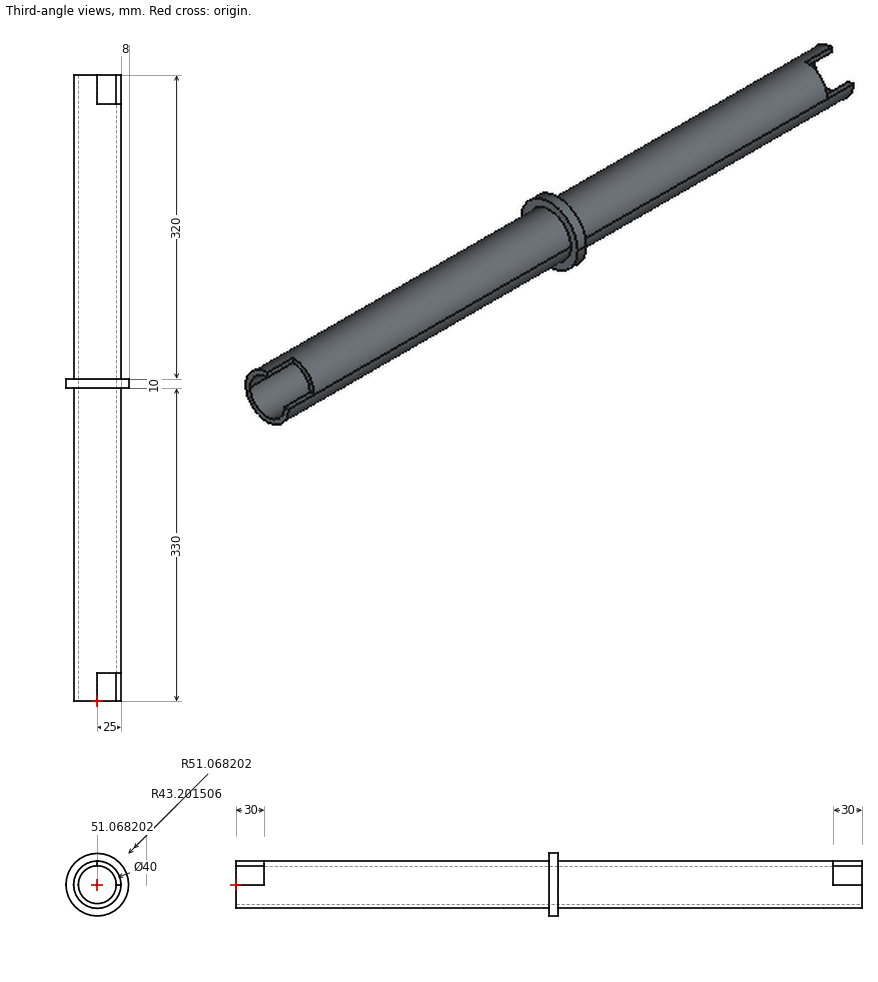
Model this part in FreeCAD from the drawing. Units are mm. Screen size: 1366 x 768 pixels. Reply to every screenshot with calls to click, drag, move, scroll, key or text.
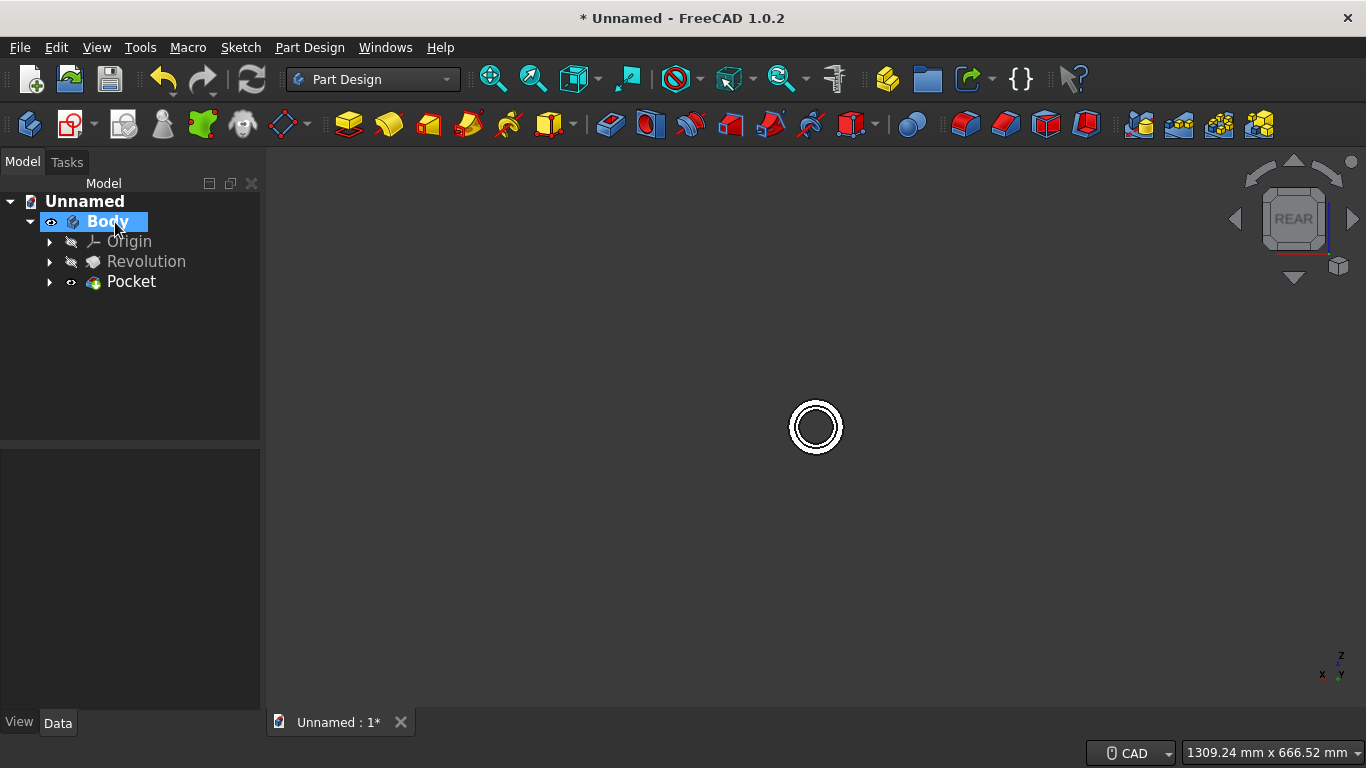
click(494, 80)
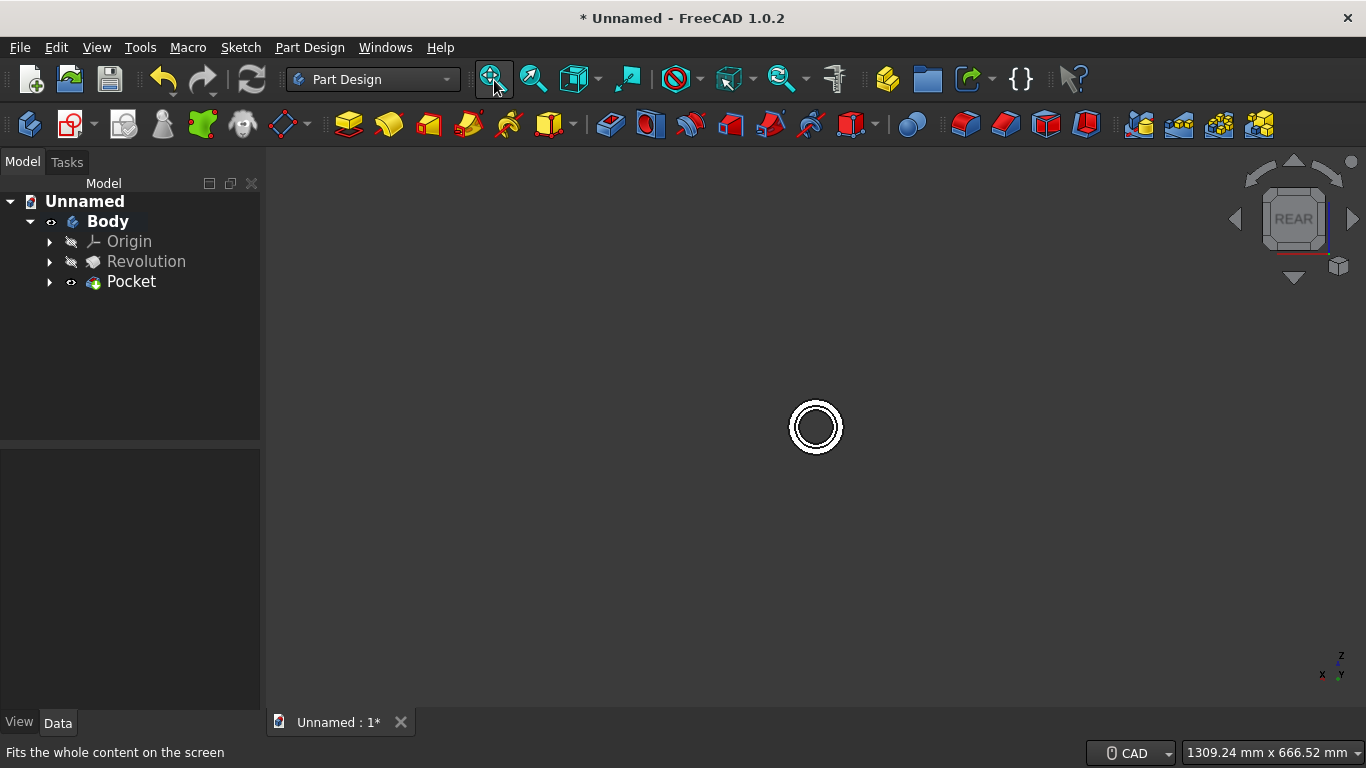
scroll(834, 432, up, 9)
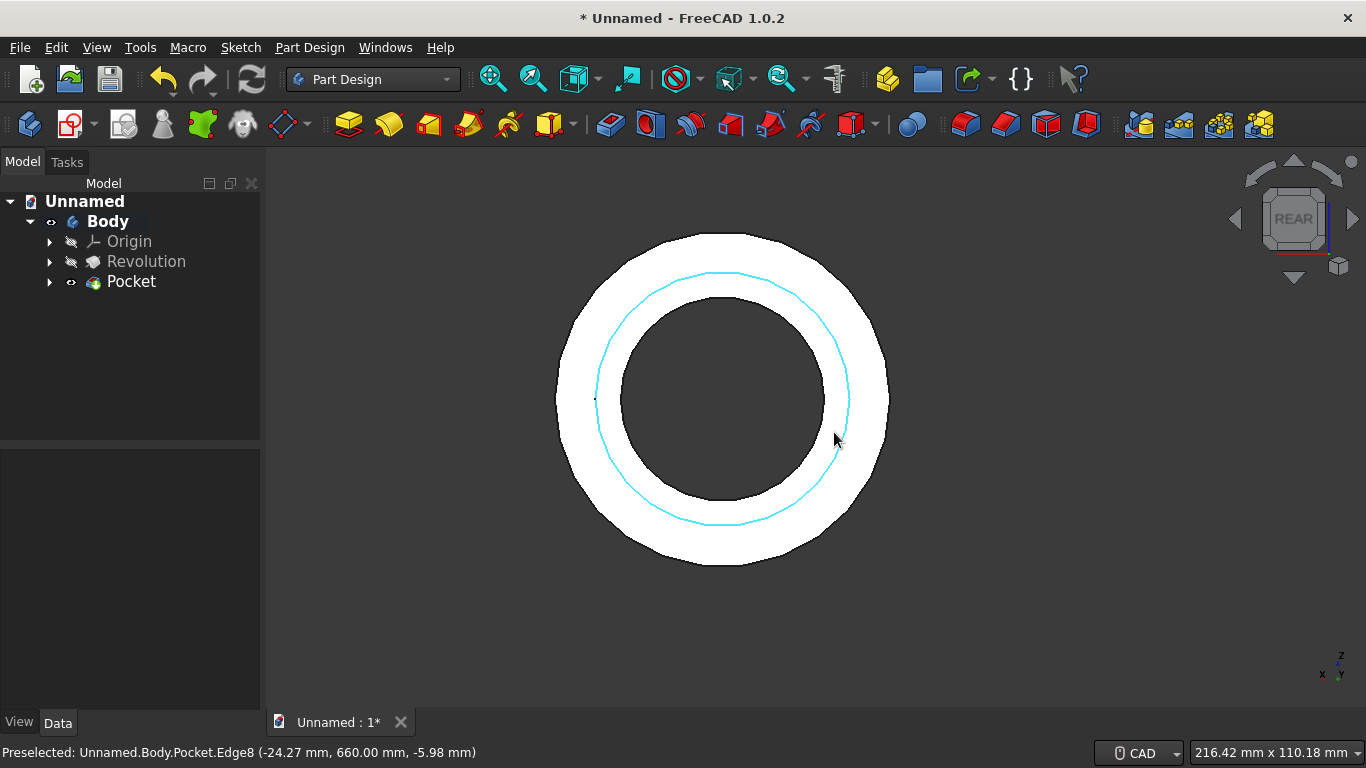
click(831, 434)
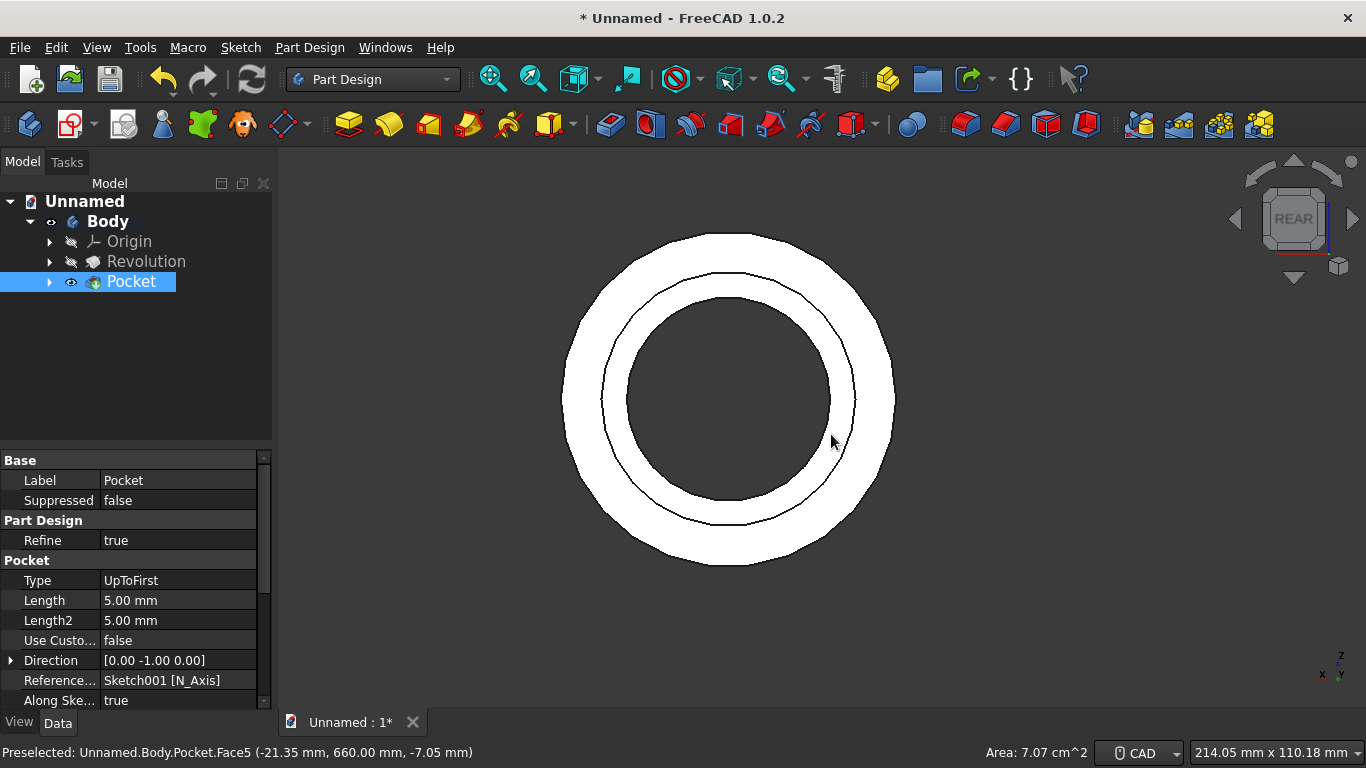
click(70, 124)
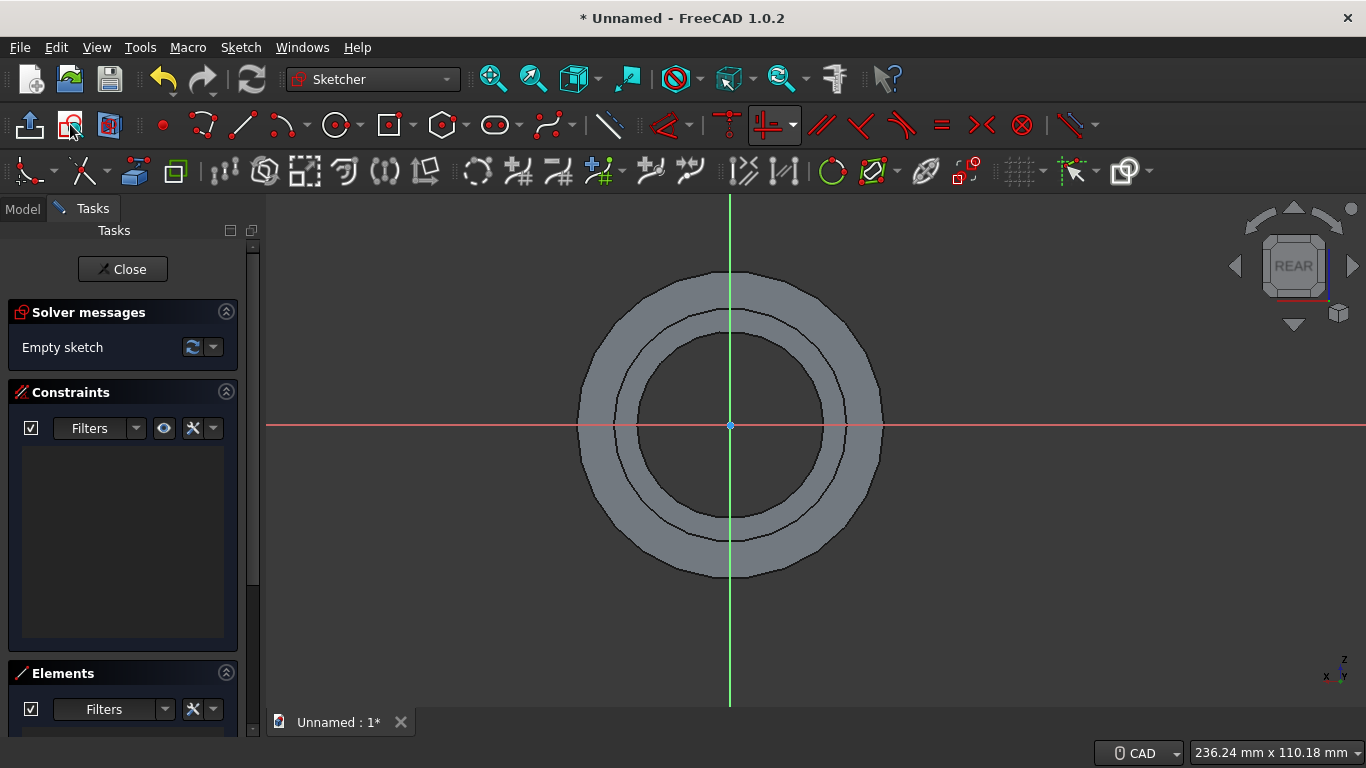
scroll(1201, 679, down, 1)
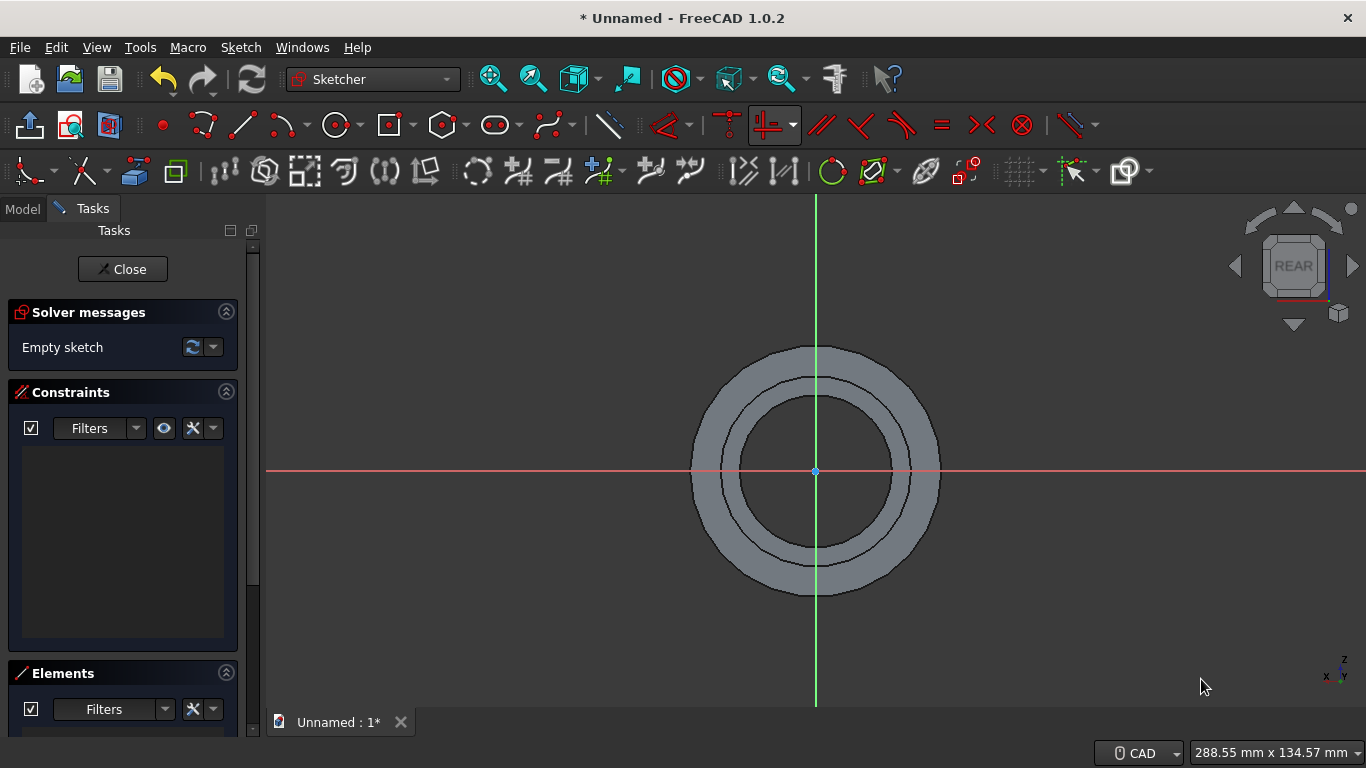
scroll(716, 314, up, 3)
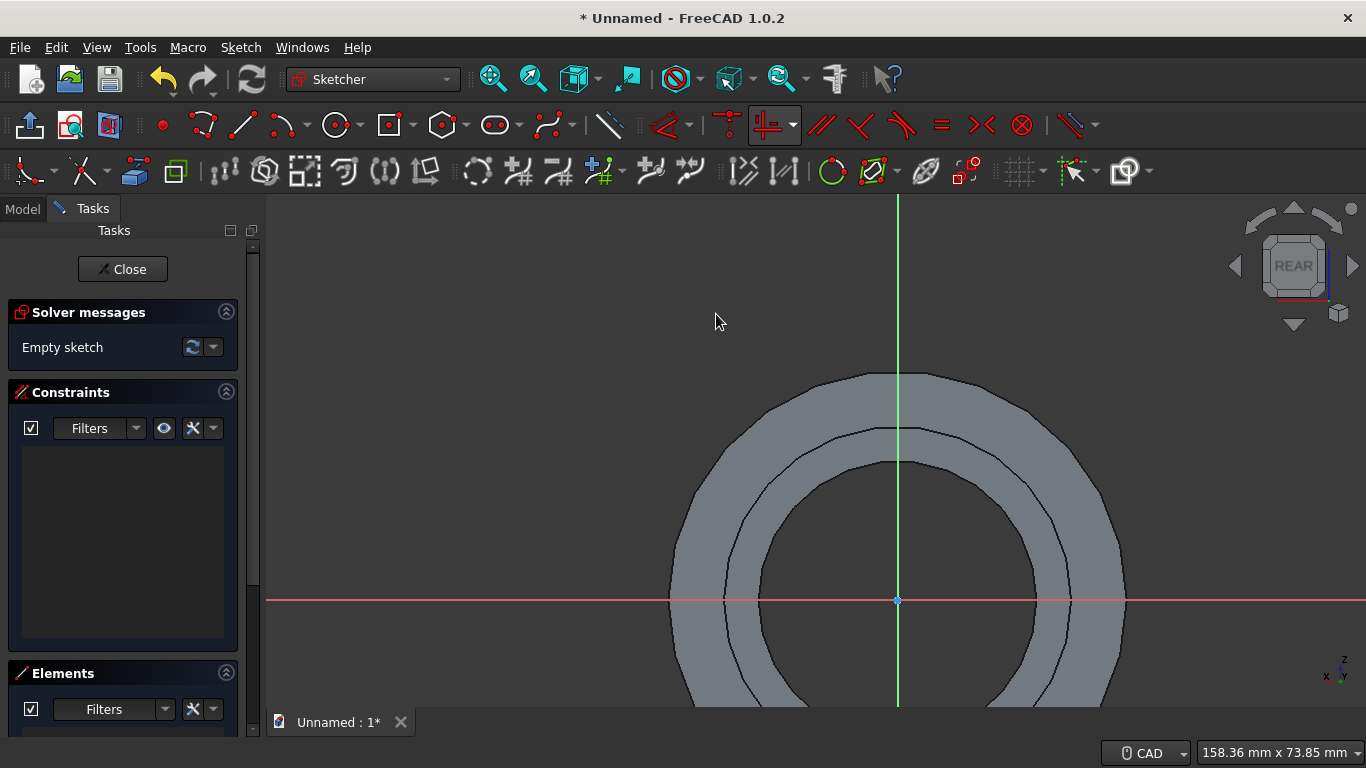
click(204, 126)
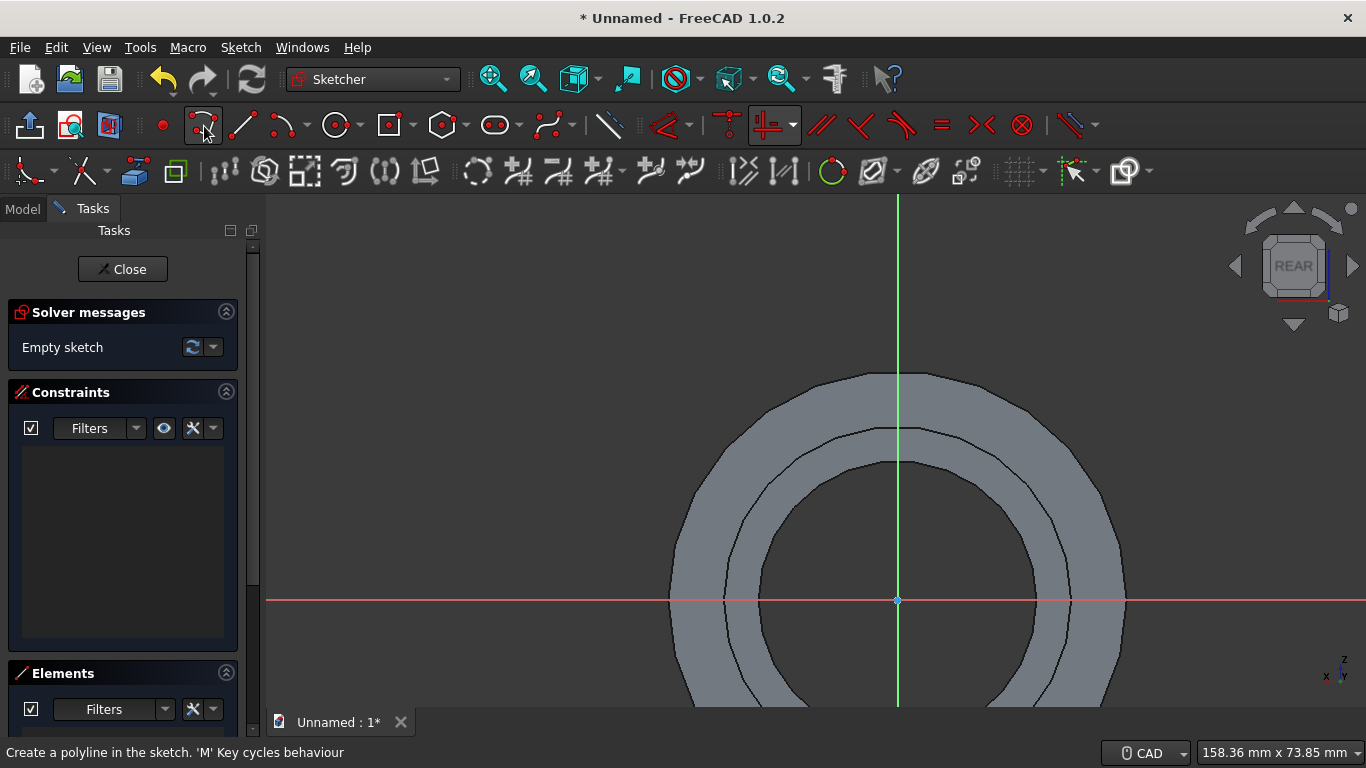
click(597, 600)
click(898, 600)
click(889, 300)
right_click(889, 300)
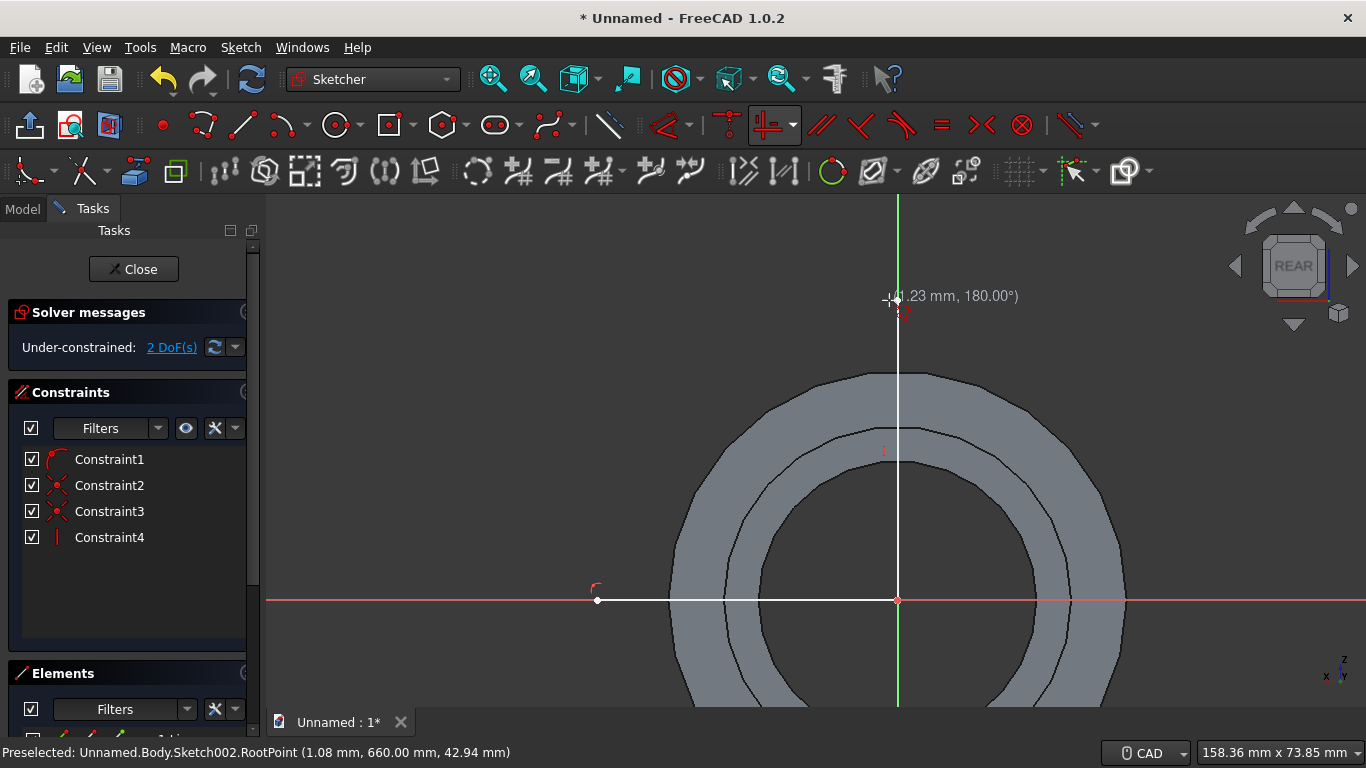
click(310, 126)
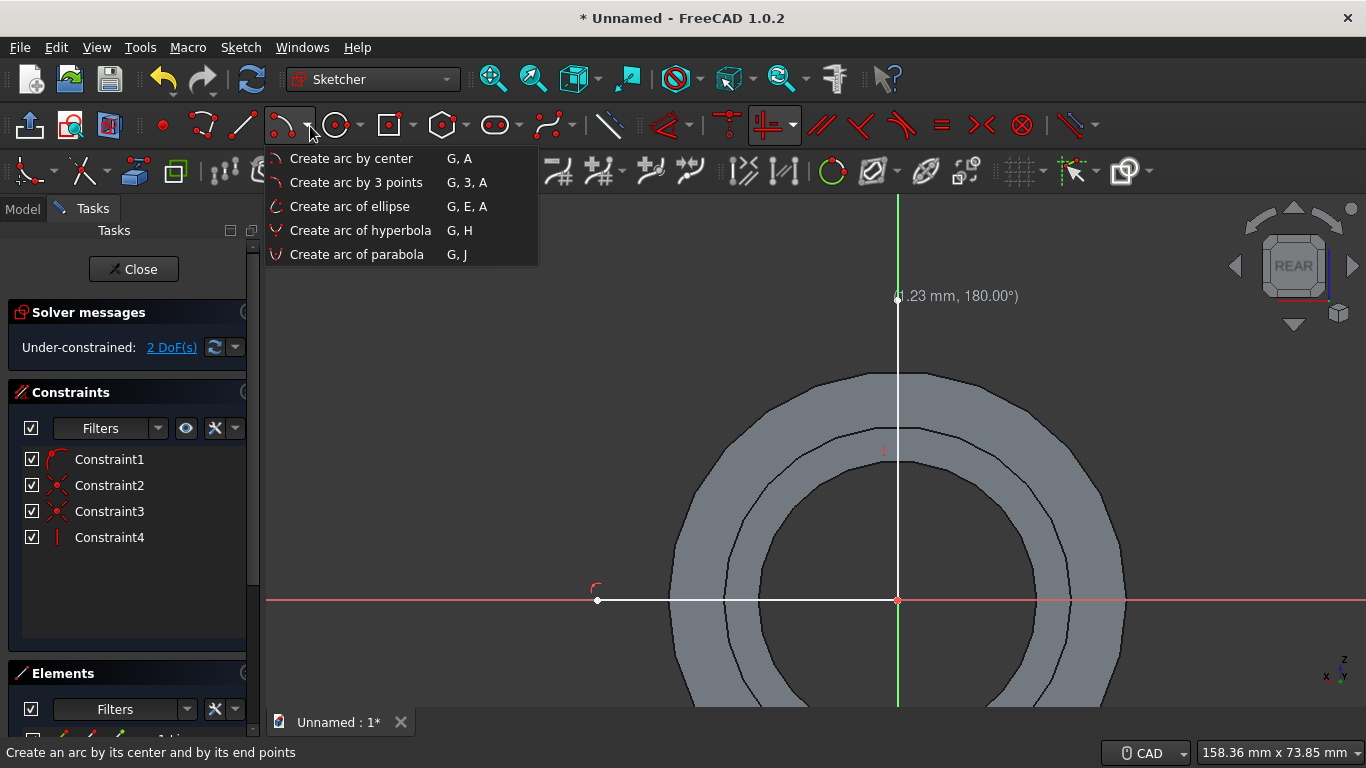
click(402, 182)